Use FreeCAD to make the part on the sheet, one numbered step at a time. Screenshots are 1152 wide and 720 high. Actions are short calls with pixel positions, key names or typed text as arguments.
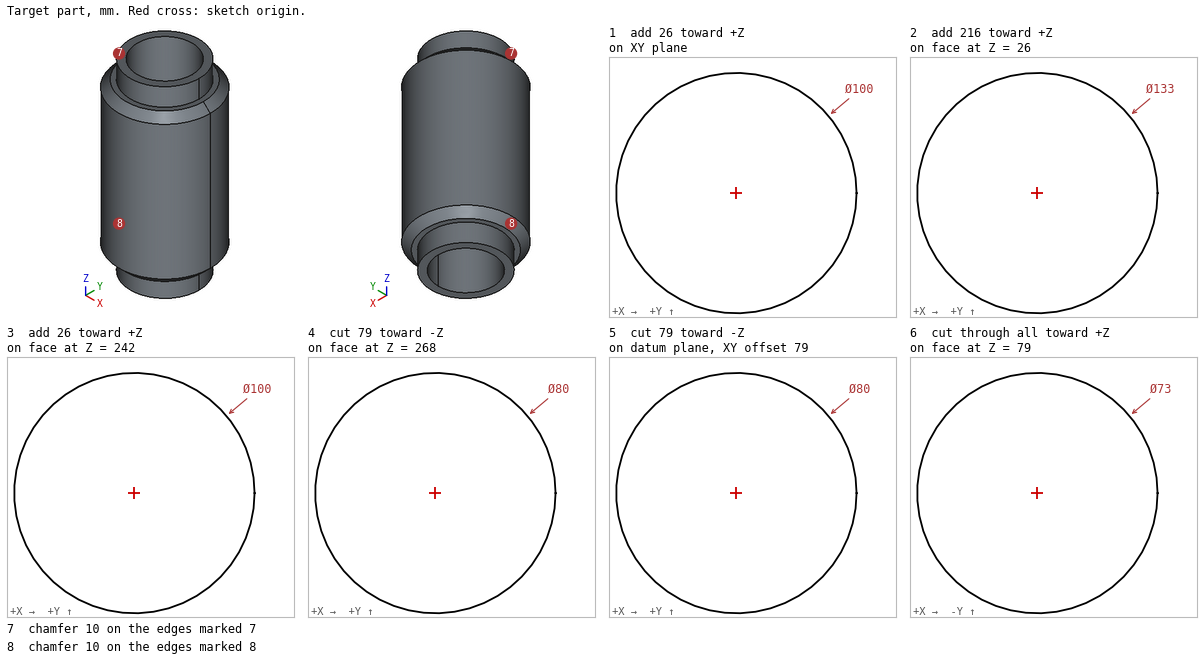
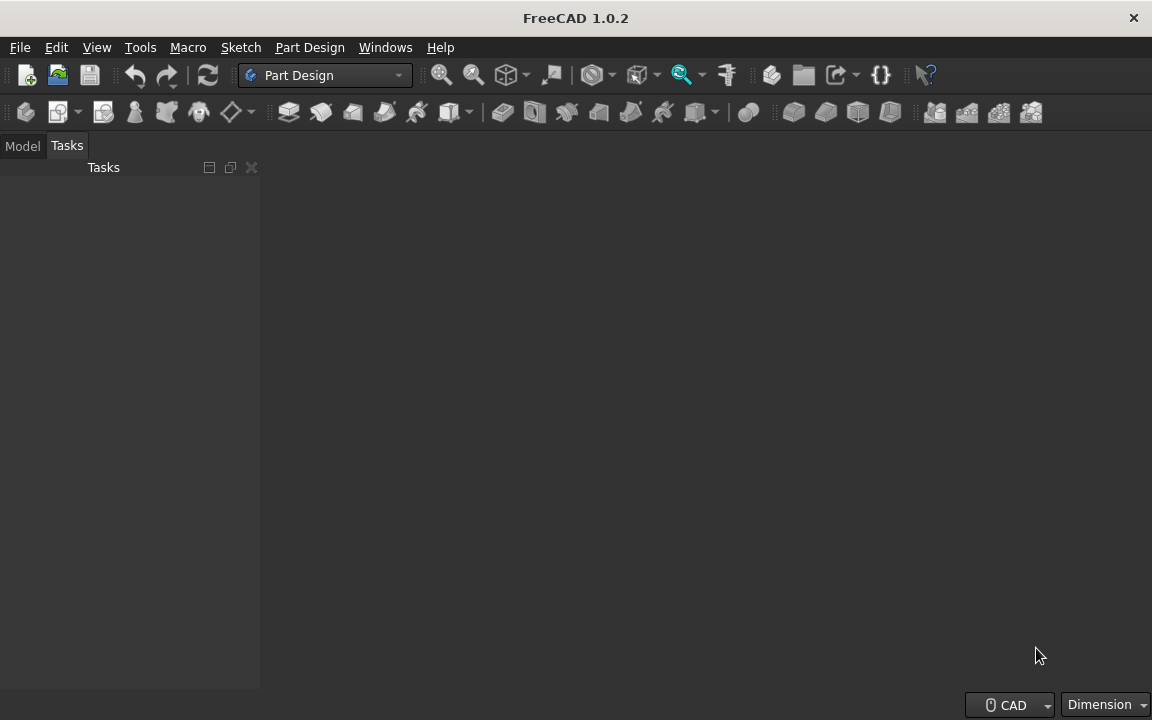
key(ctrl+n)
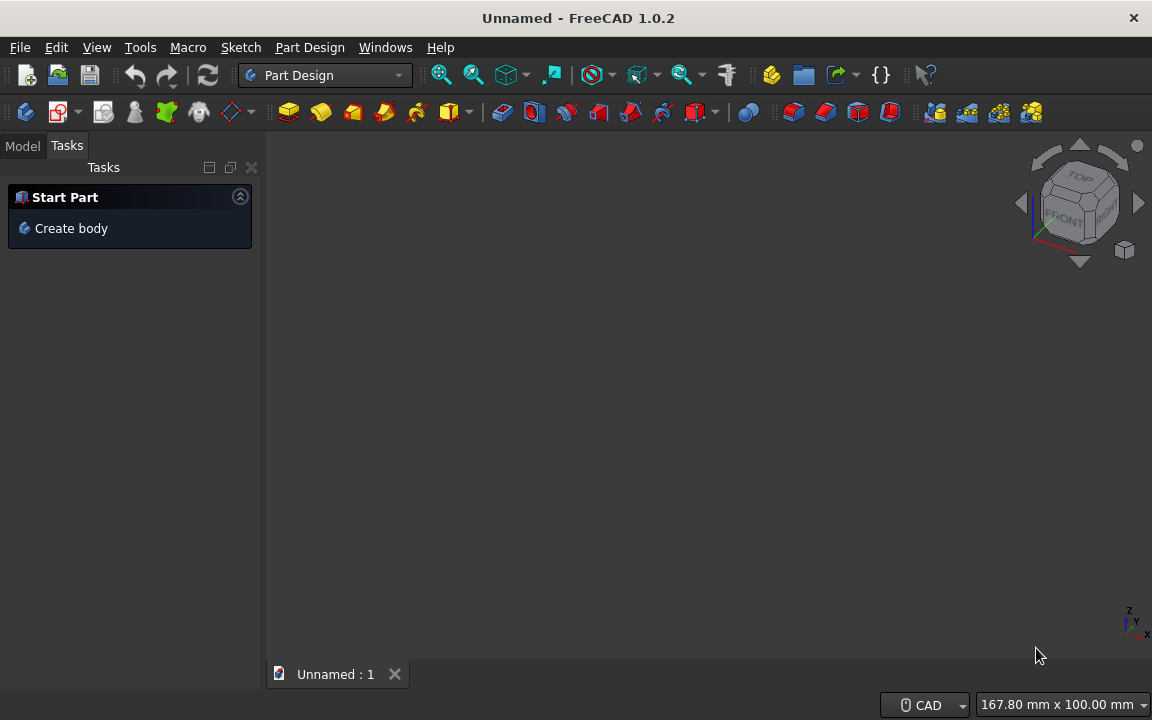
click(58, 112)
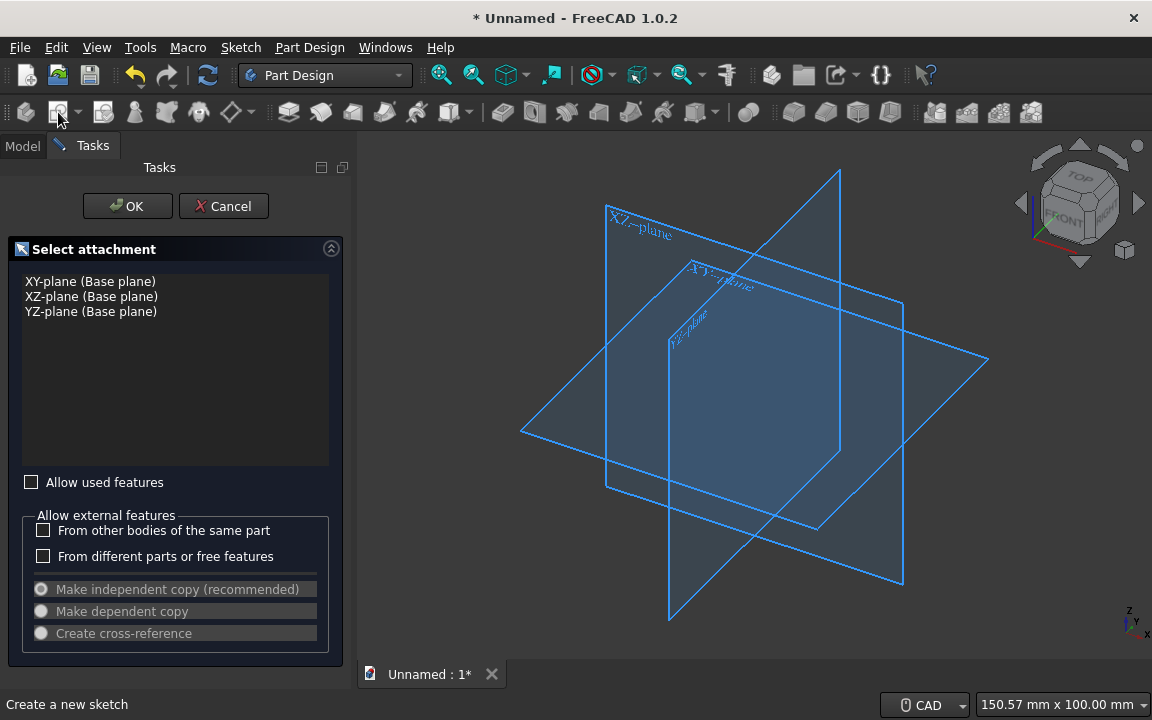
click(82, 282)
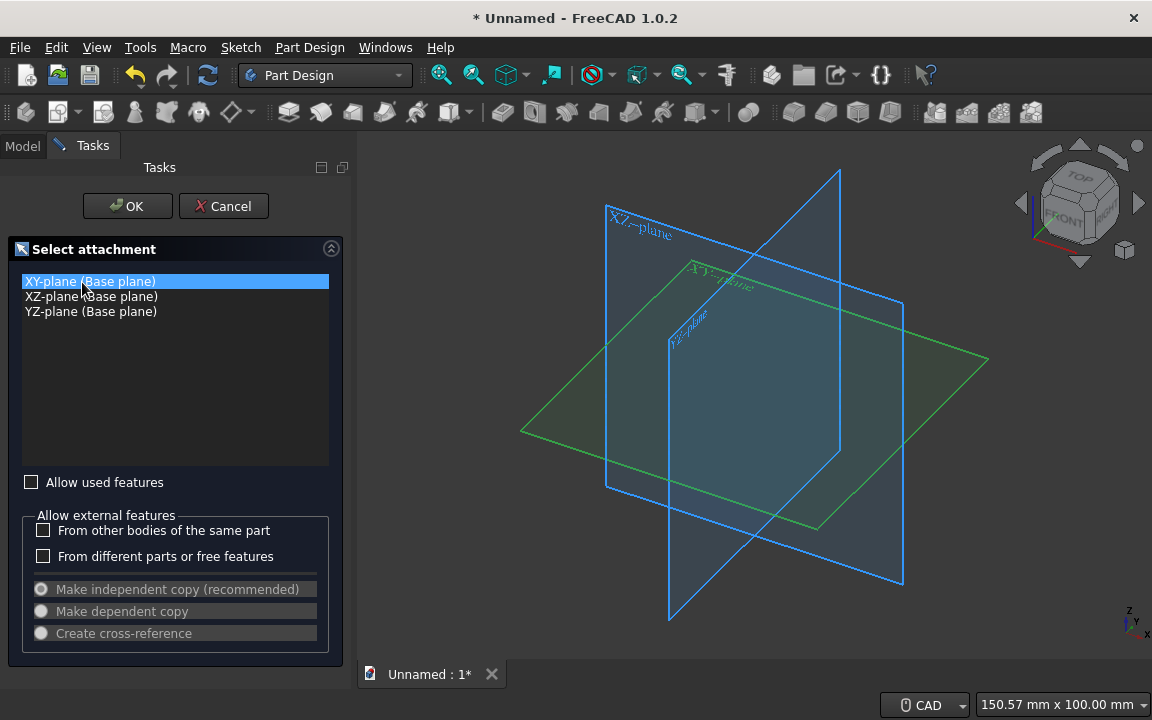
click(128, 206)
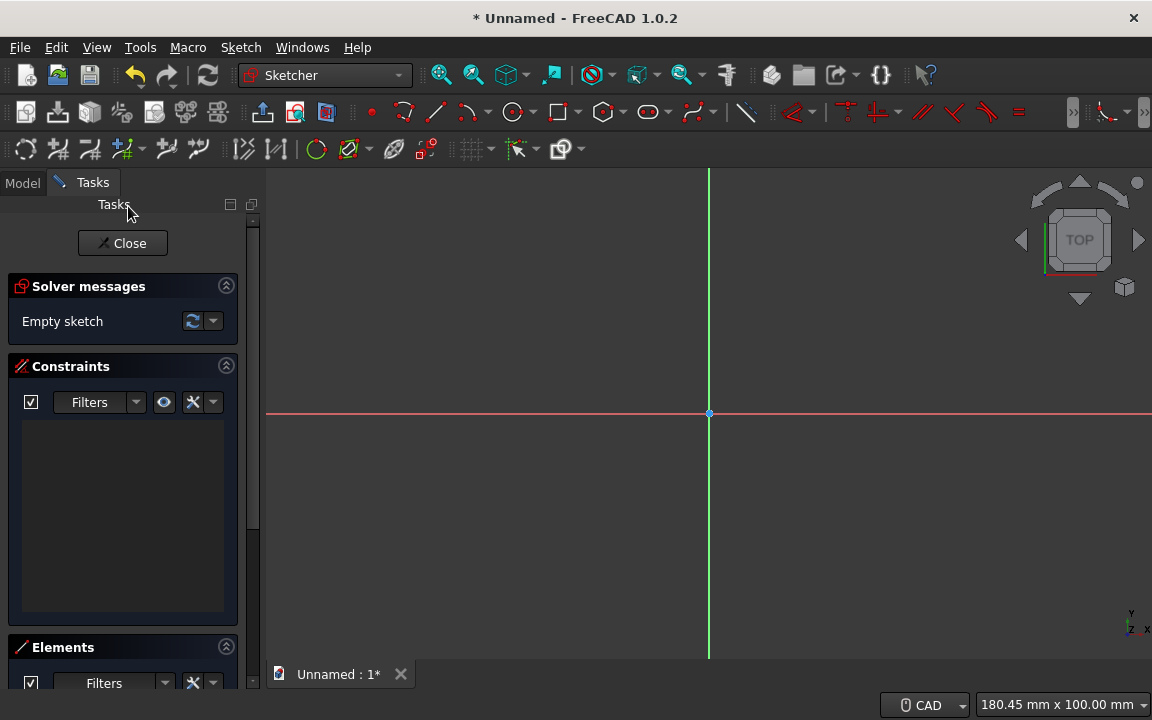
scroll(501, 414, down, 2)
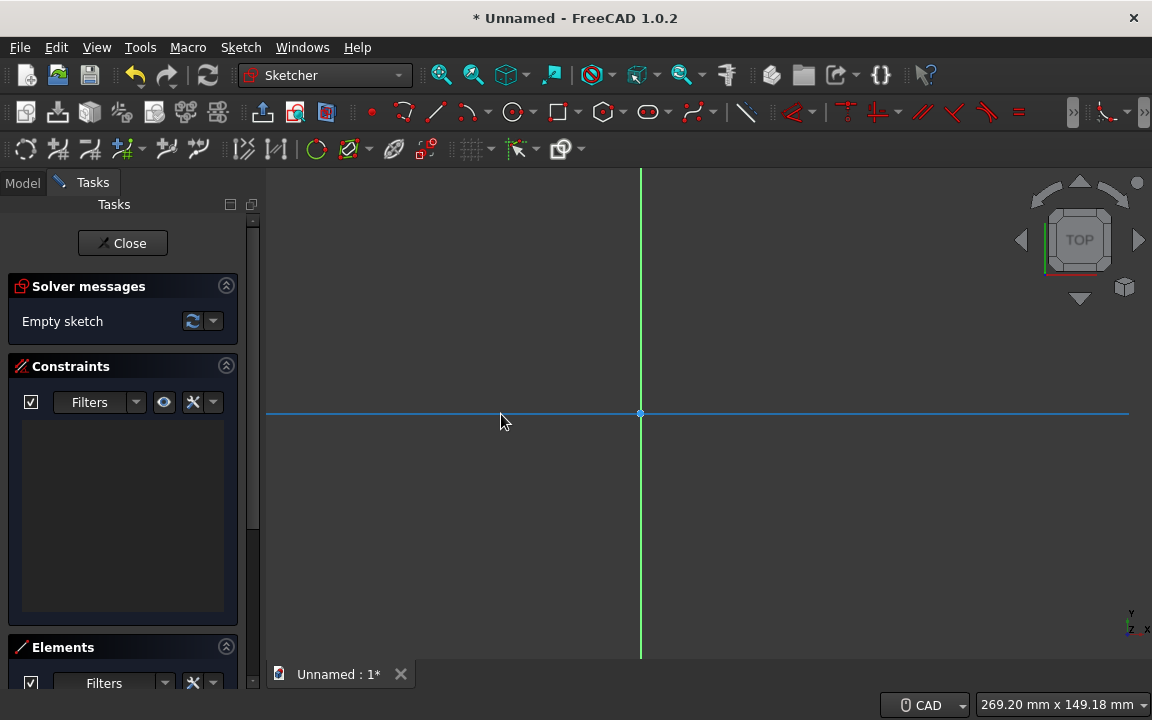
key(g)
key(c)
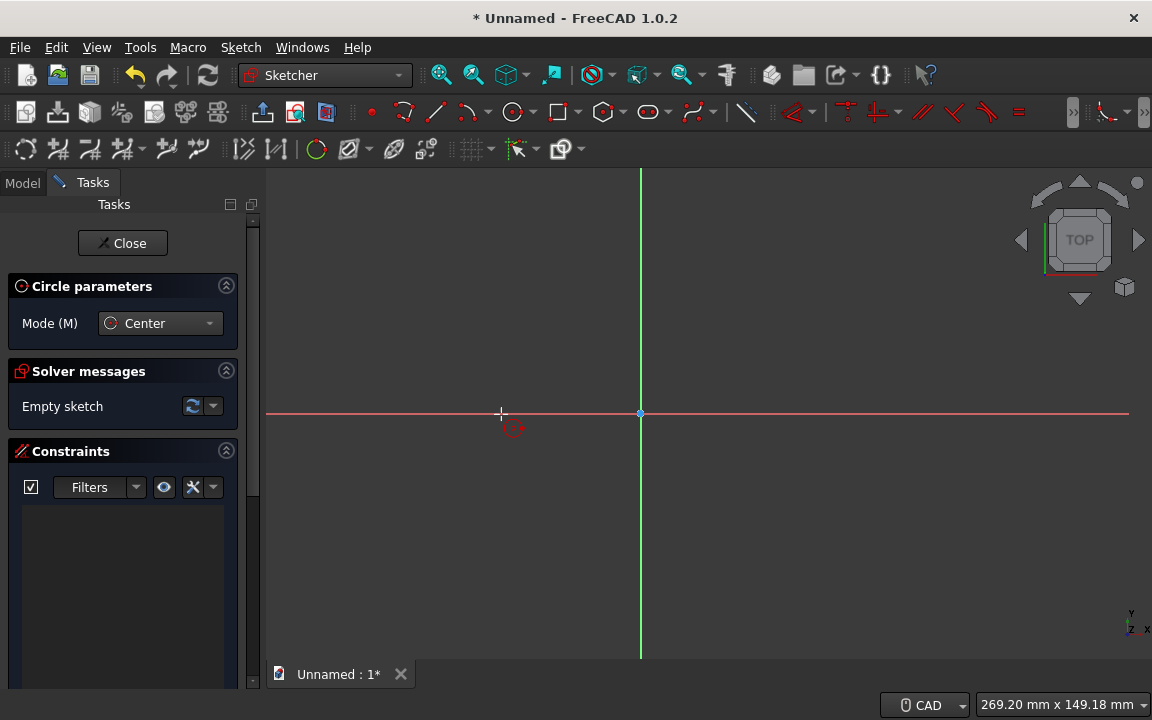
click(641, 414)
move(757, 297)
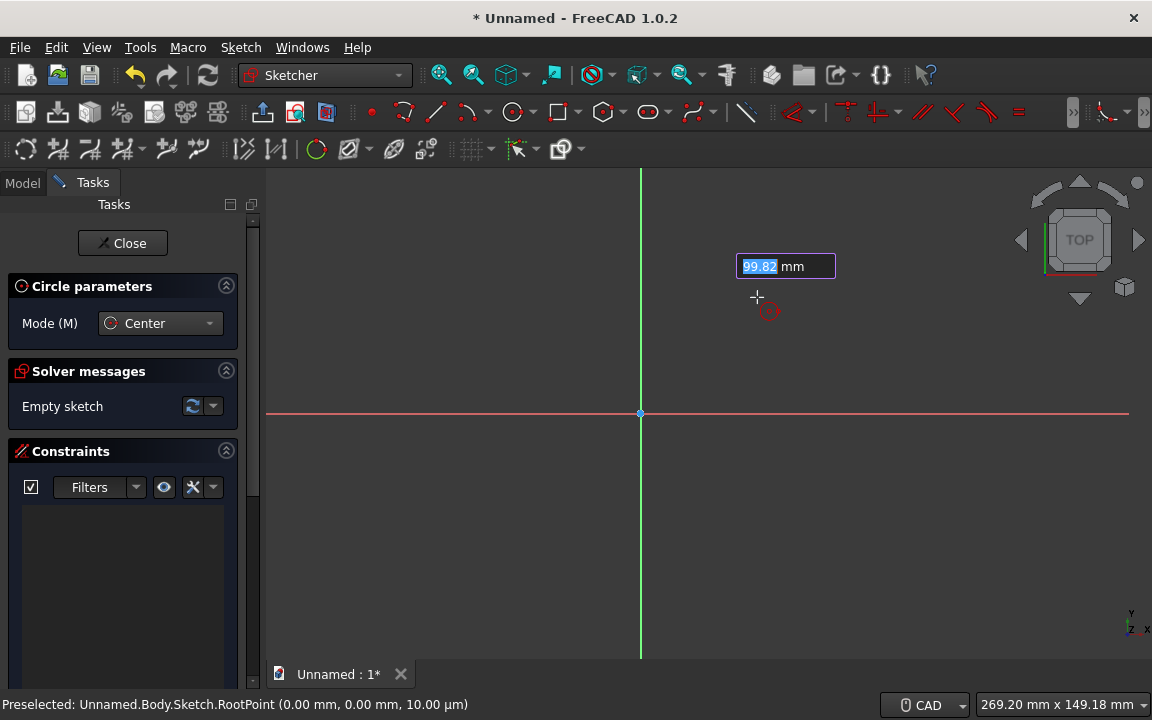
text(100)
key(Return)
key(Escape)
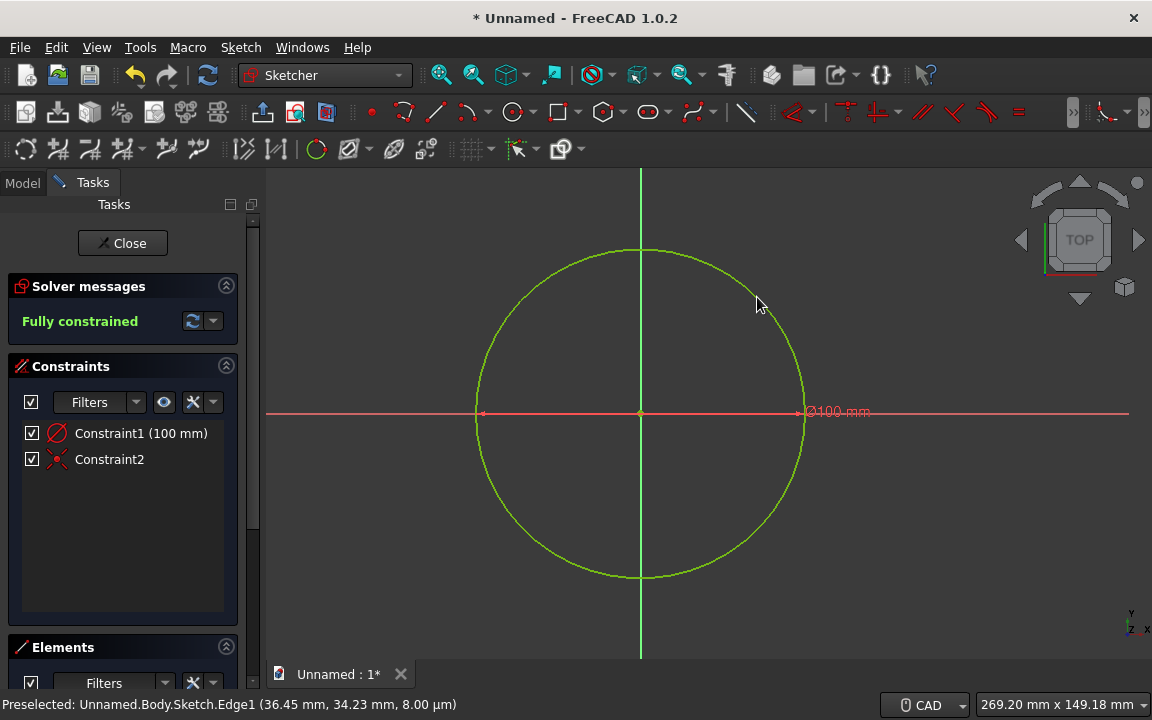
click(123, 243)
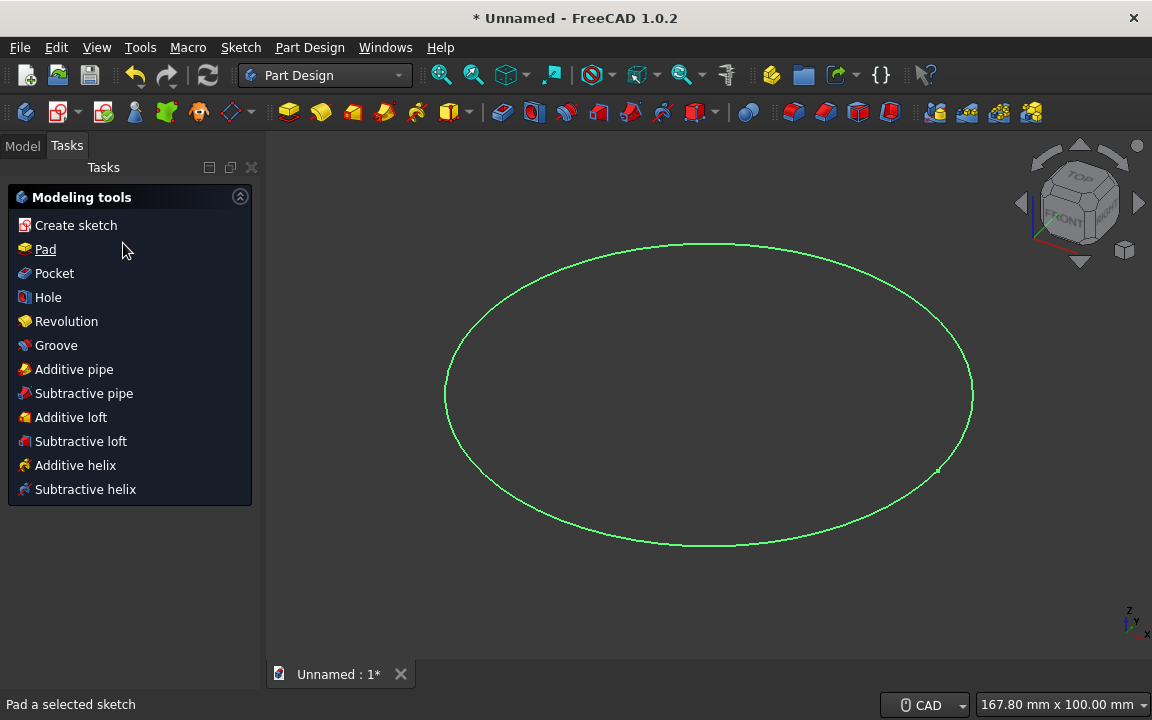
click(290, 112)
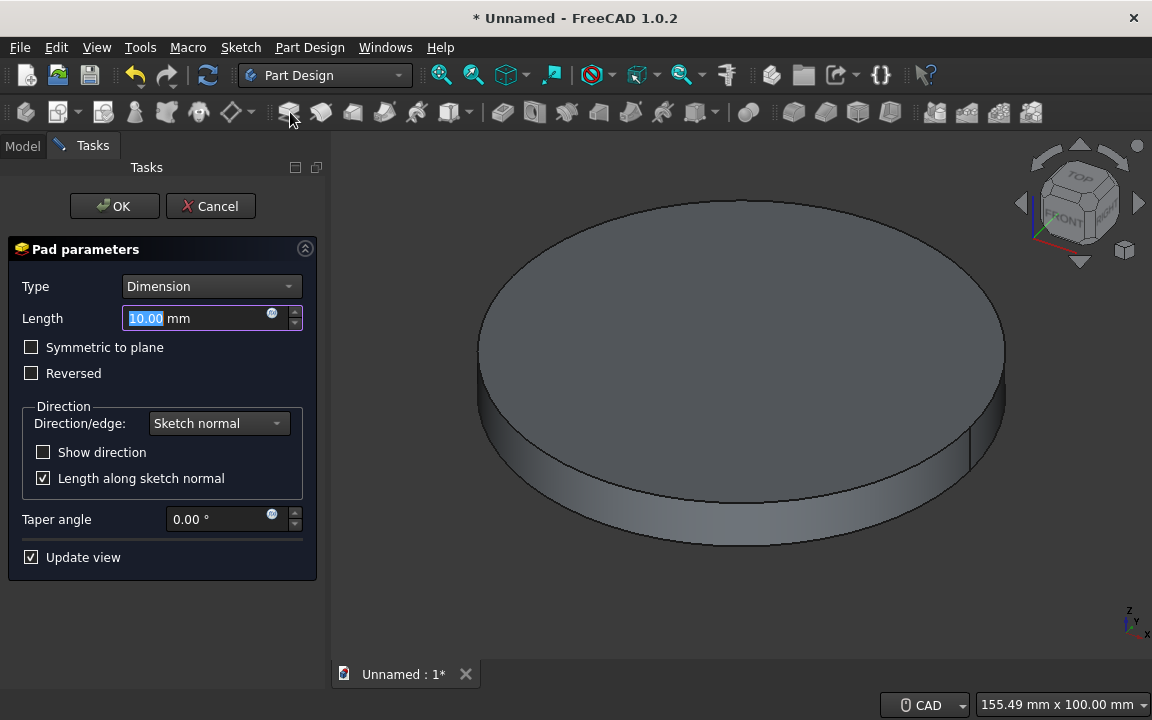
text(26)
key(Tab)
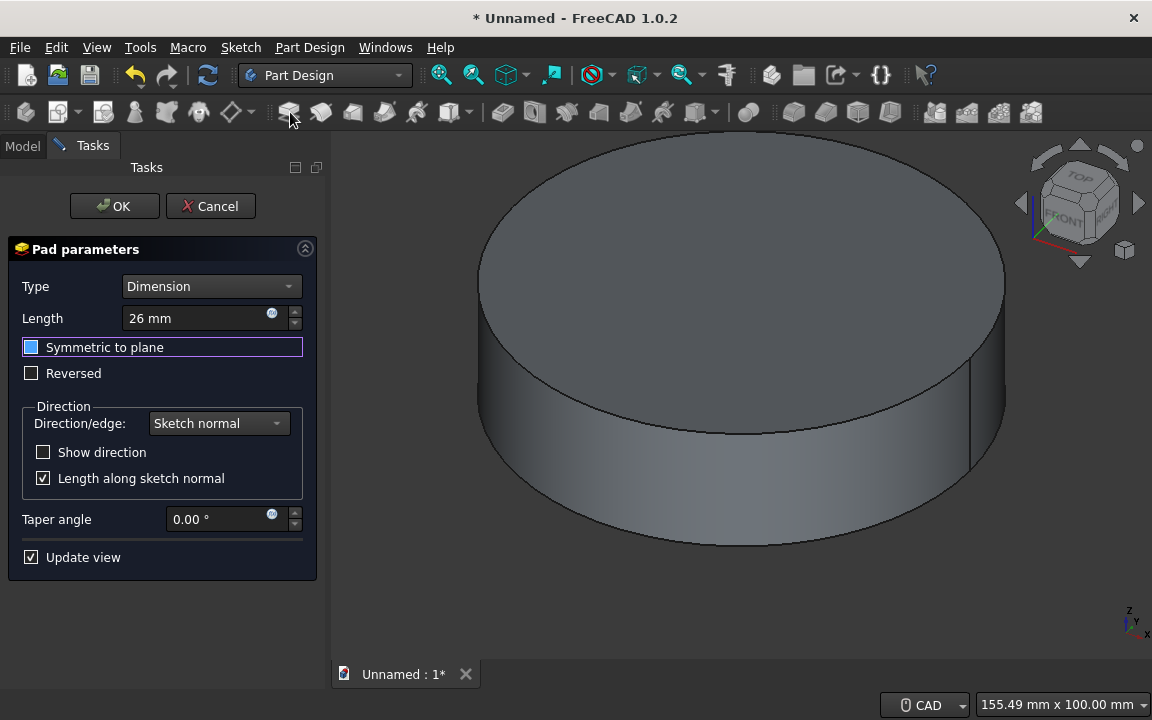
click(115, 206)